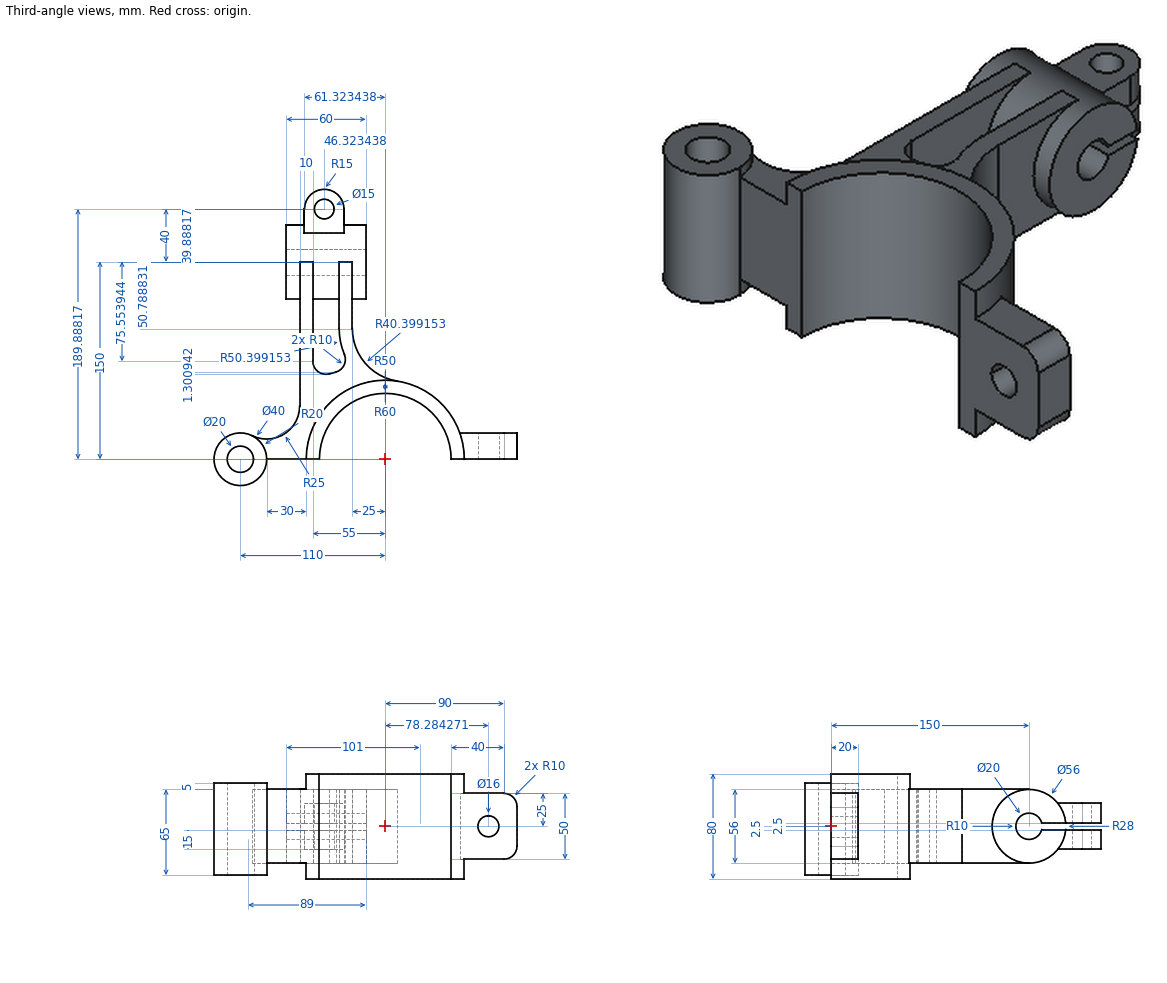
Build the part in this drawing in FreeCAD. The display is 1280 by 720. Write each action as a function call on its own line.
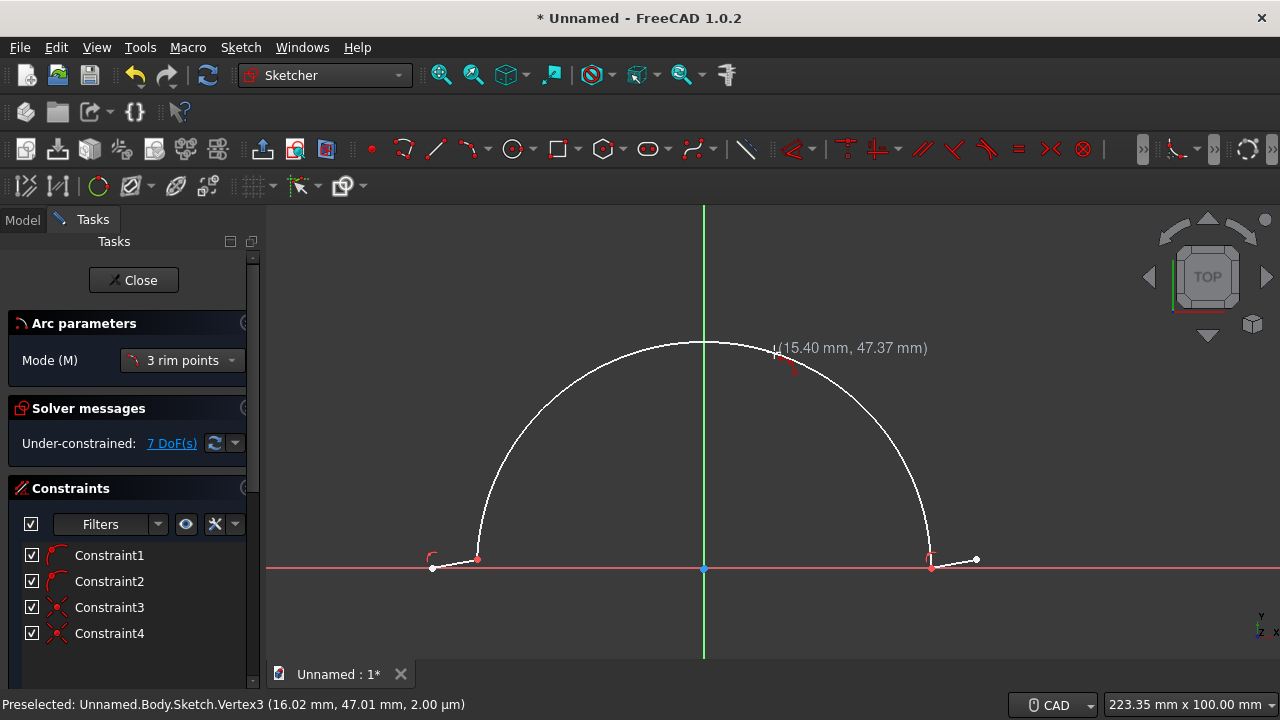
click(976, 560)
click(432, 568)
click(788, 309)
key(Escape)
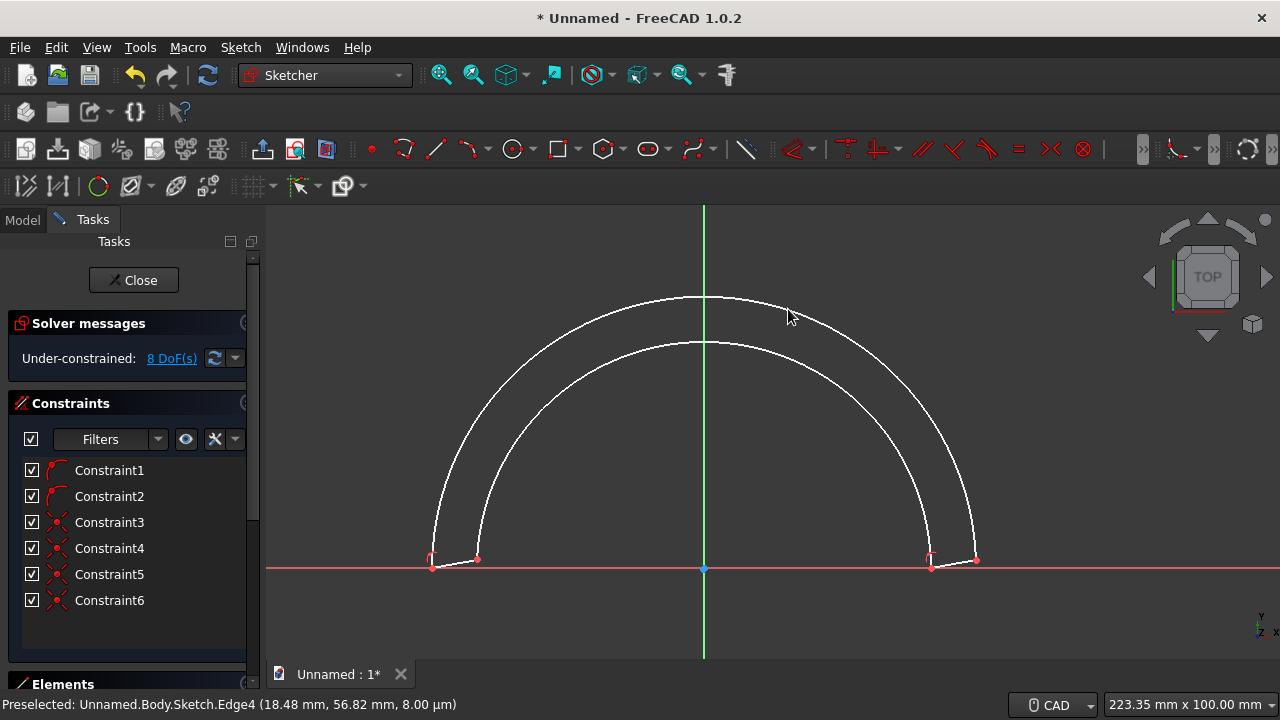
click(446, 566)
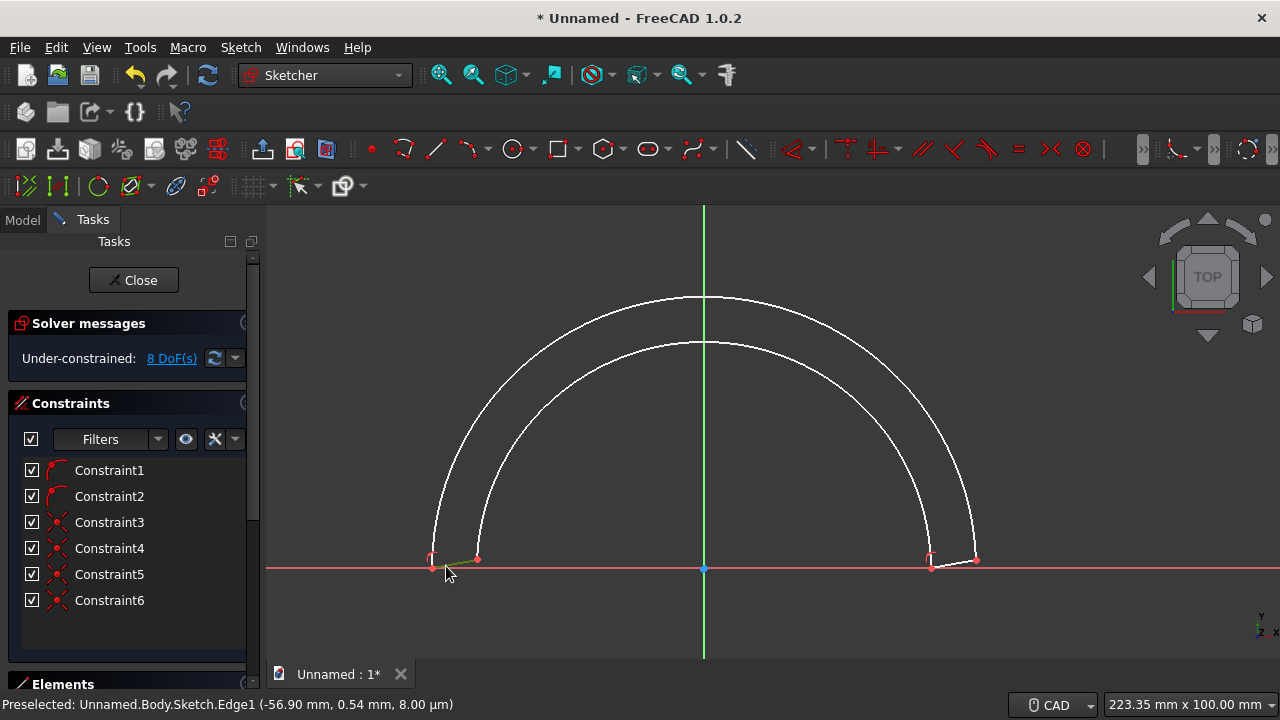
key(h)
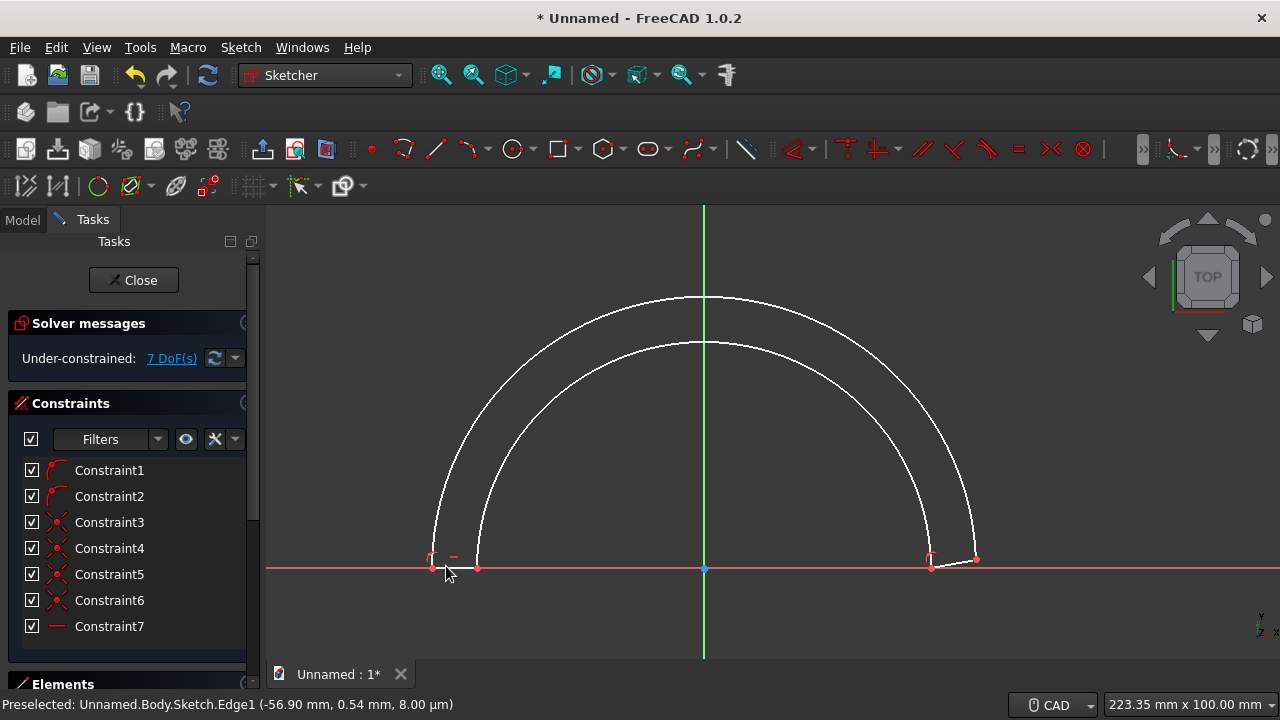
click(944, 566)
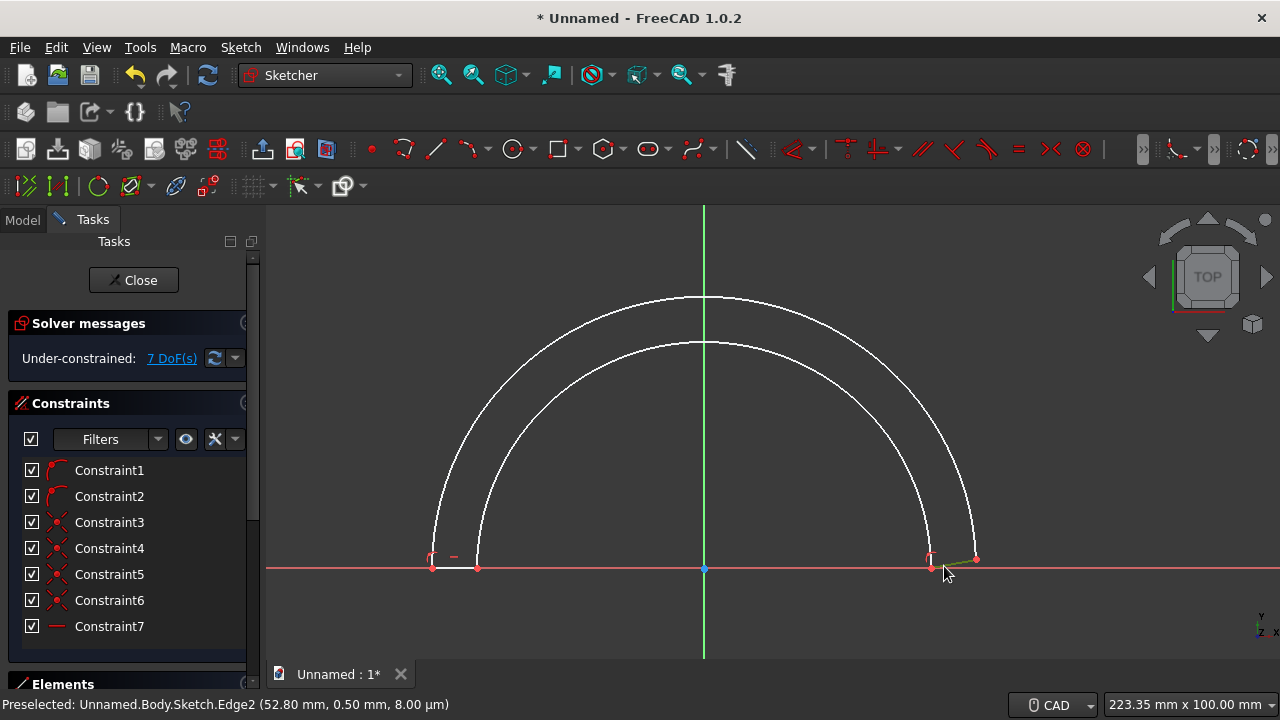
key(h)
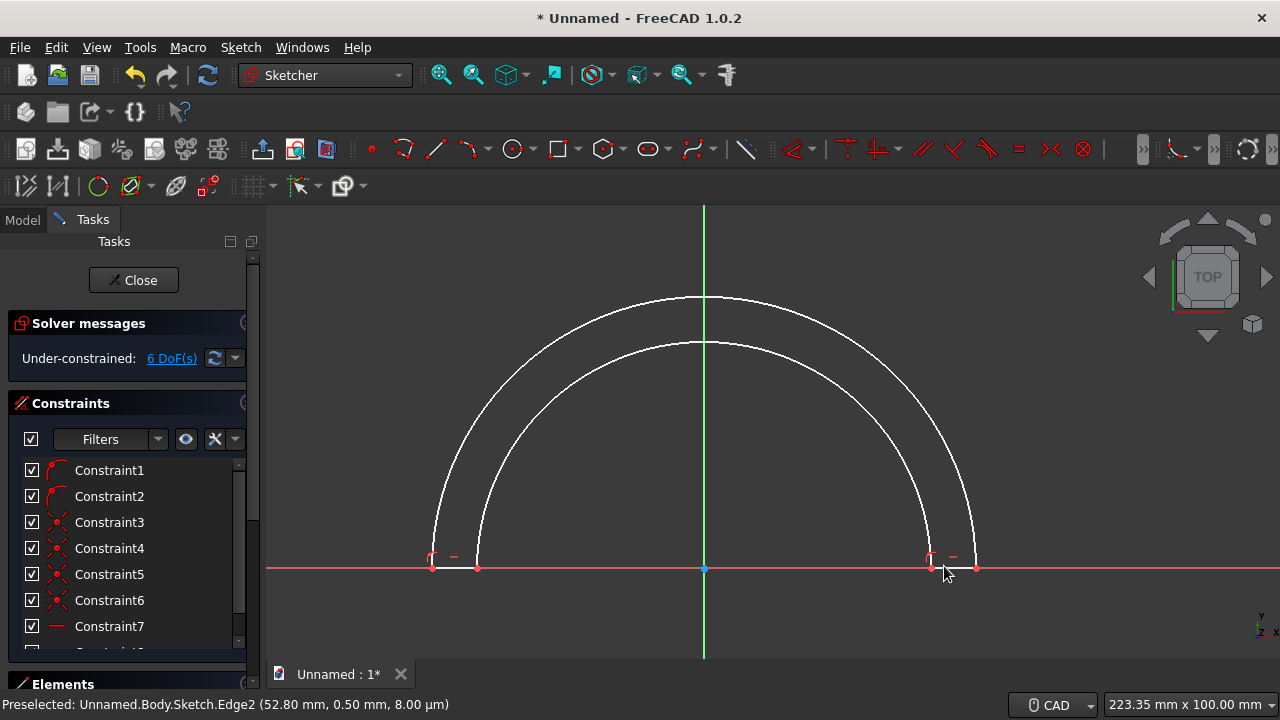
click(837, 385)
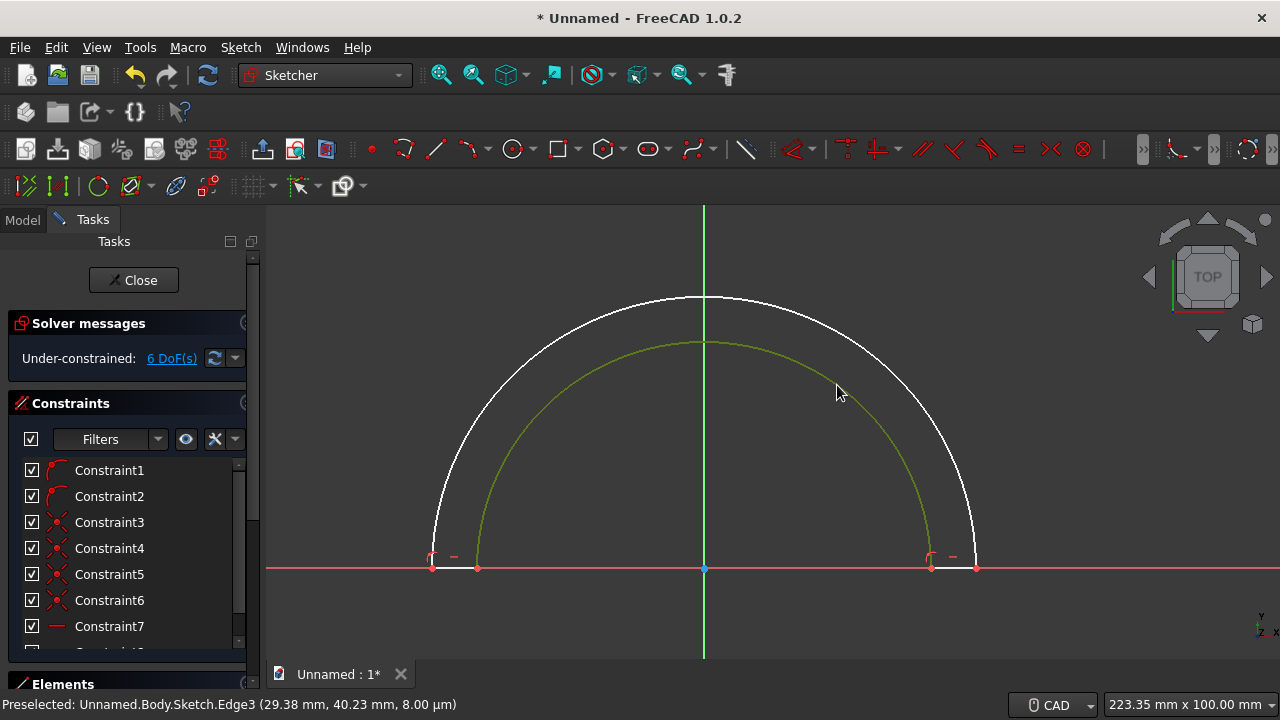
click(864, 349)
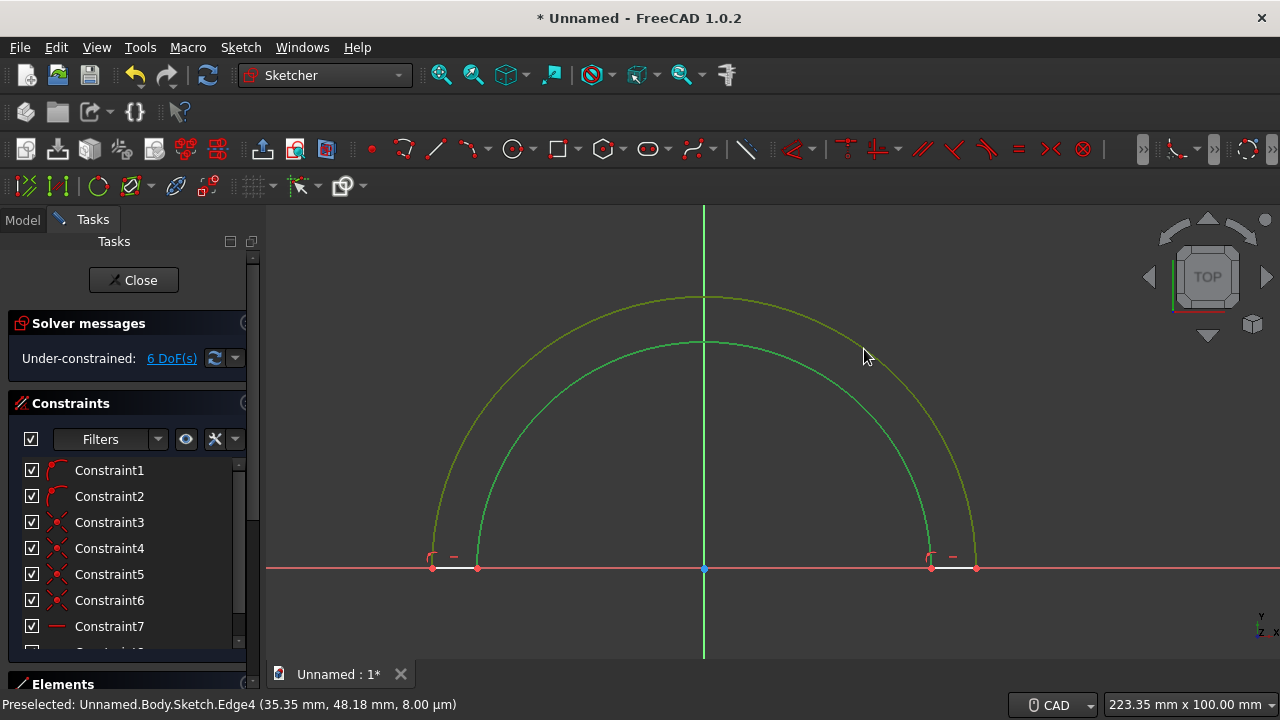
key(c)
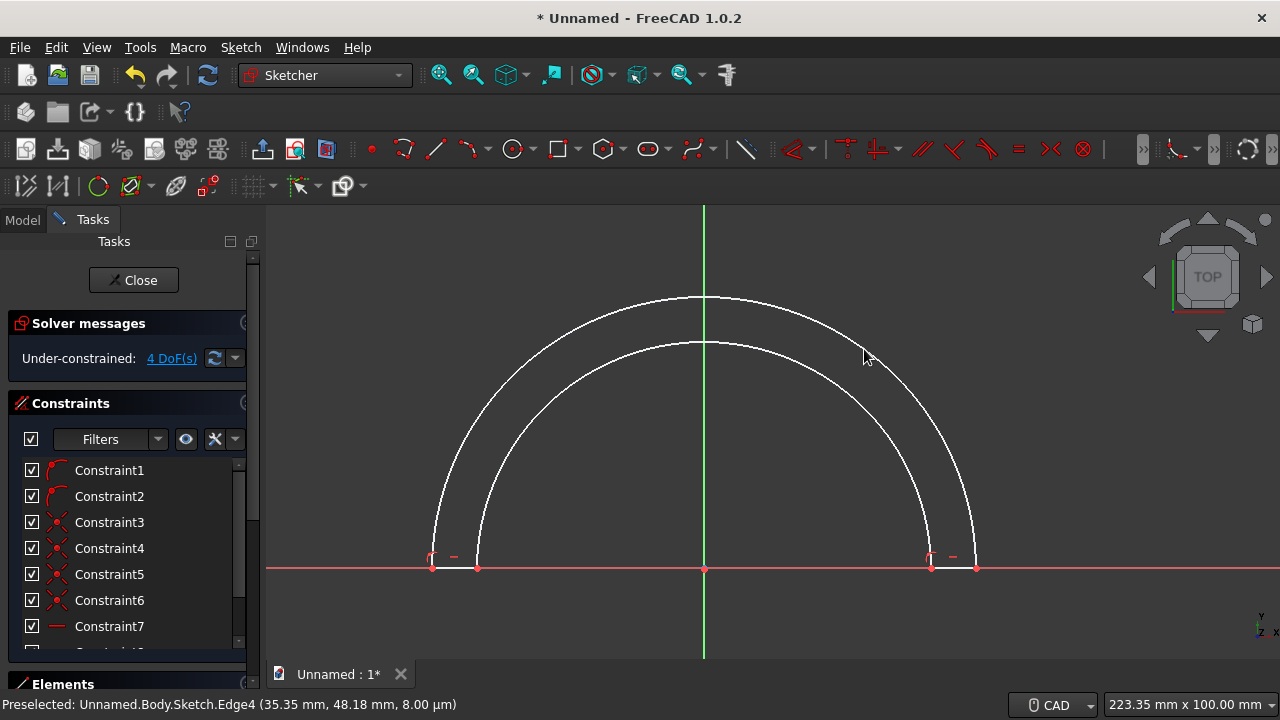
drag(694, 558, 714, 579)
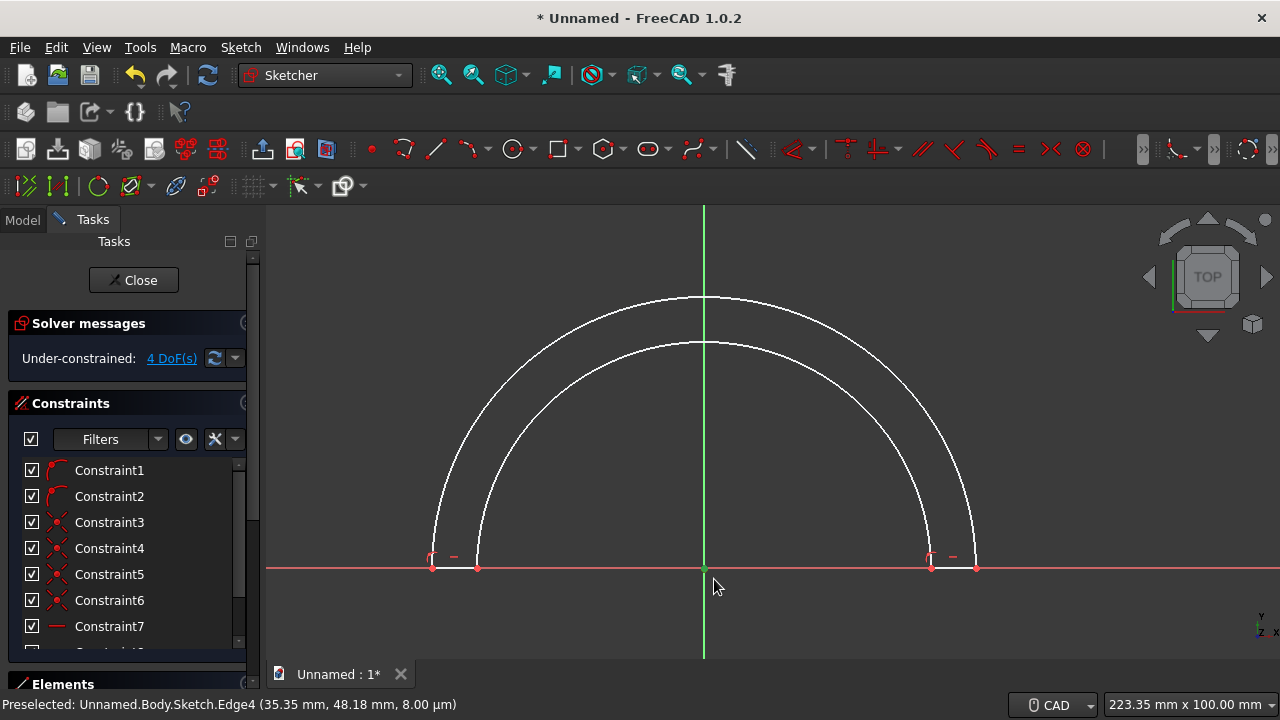
key(c)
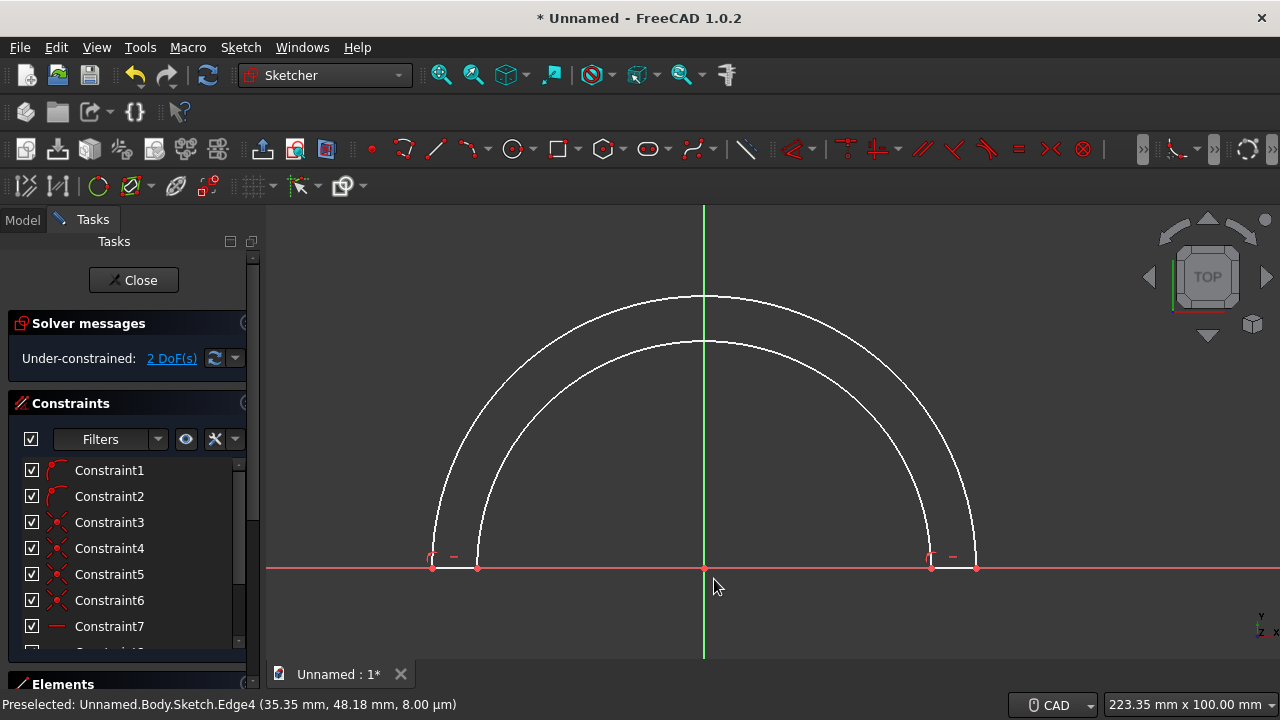
key(d)